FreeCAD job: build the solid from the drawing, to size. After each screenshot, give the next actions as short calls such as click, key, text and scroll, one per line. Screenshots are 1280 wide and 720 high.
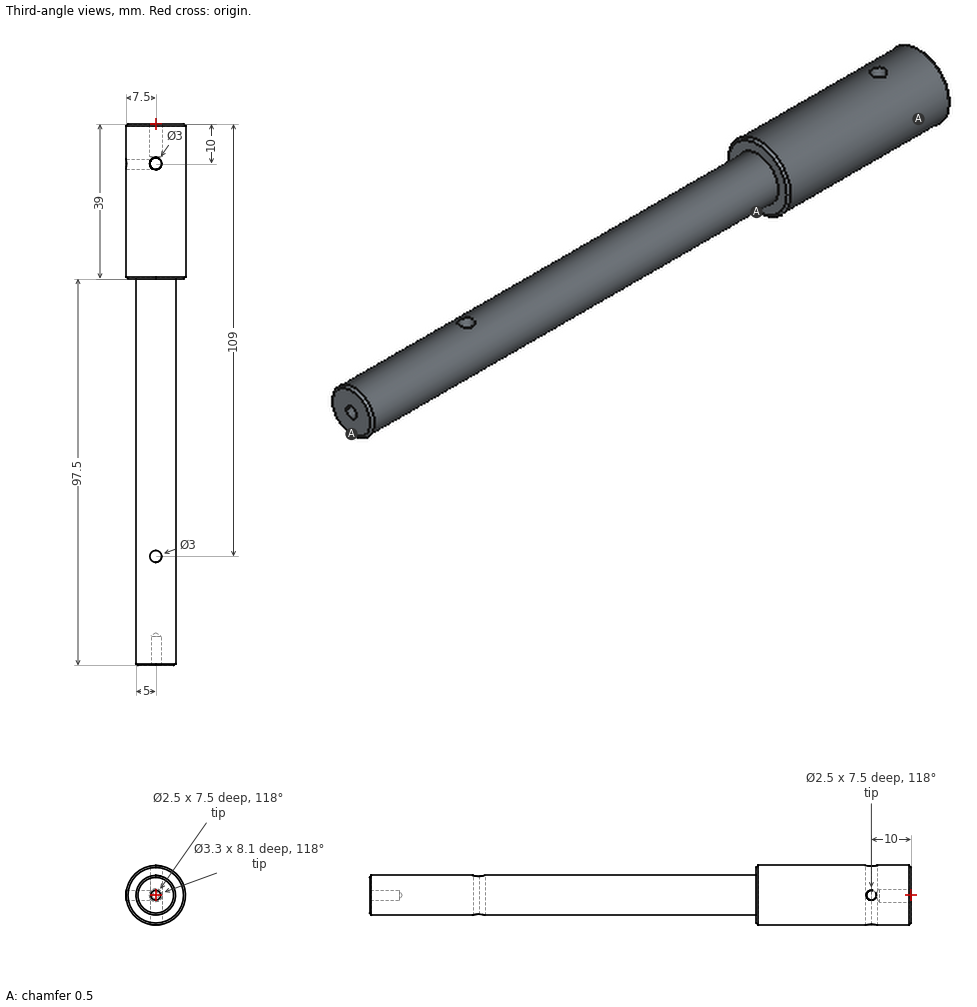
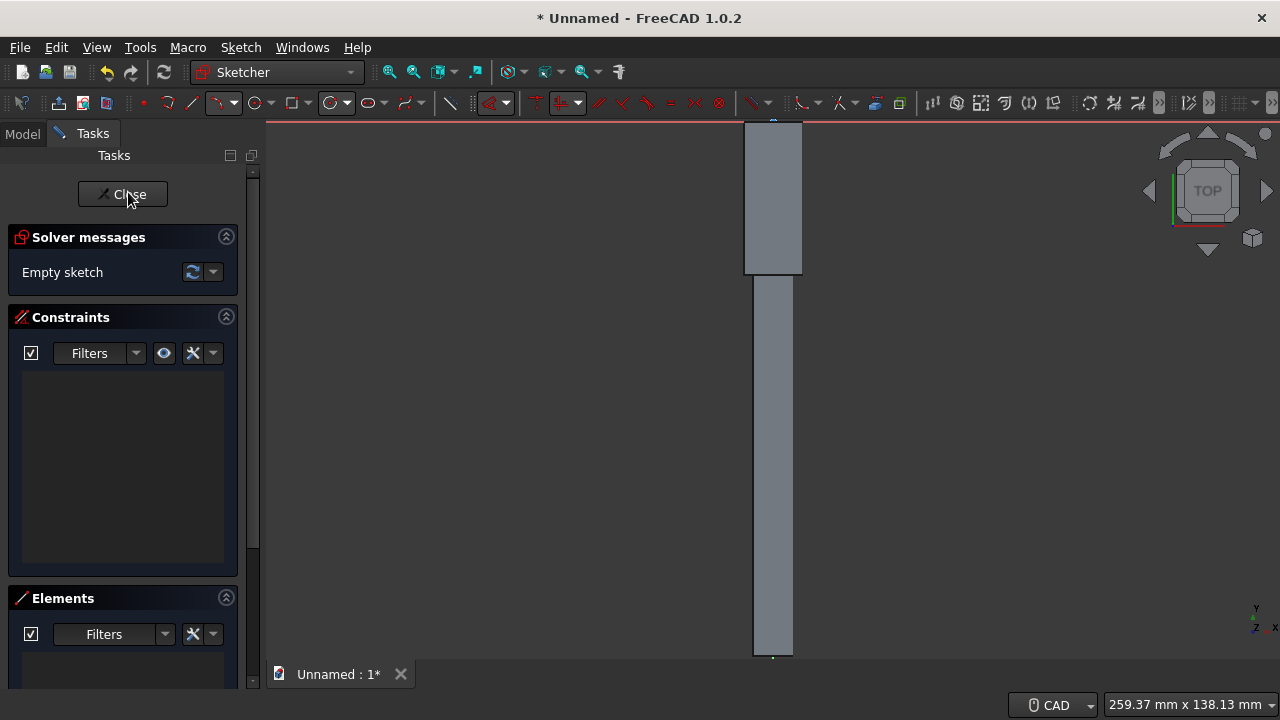
click(108, 104)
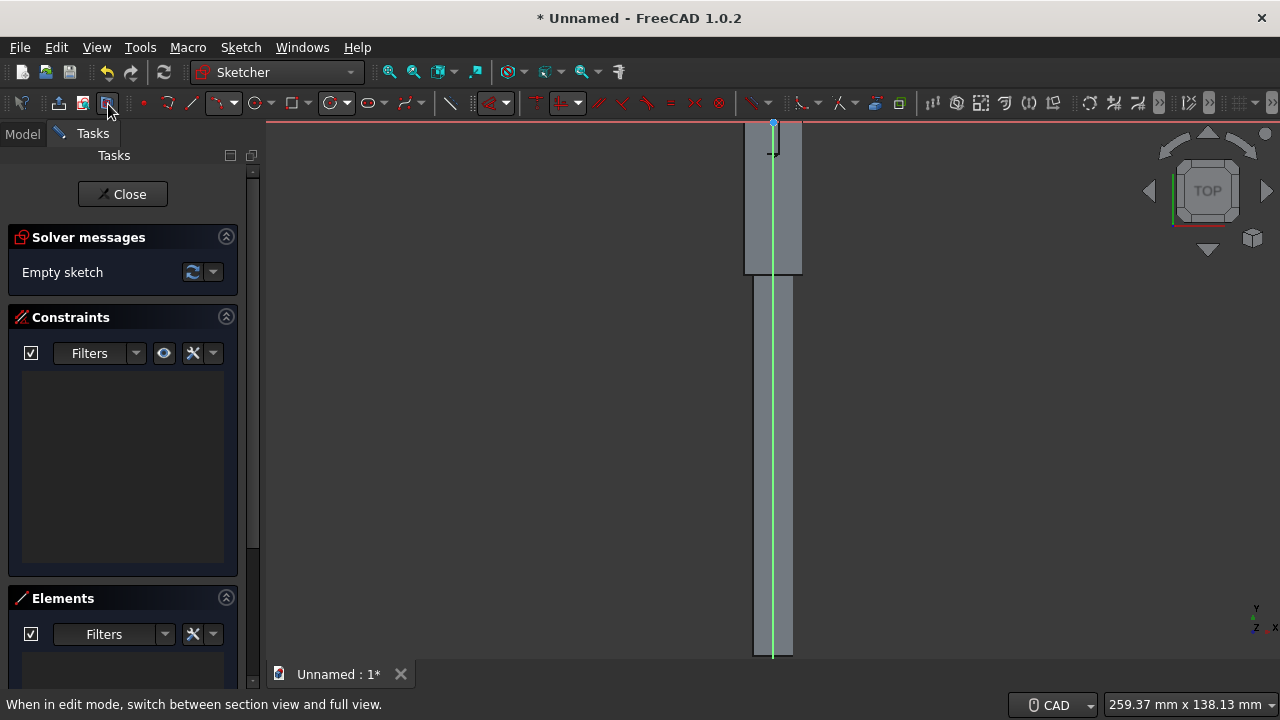
scroll(777, 149, up, 15)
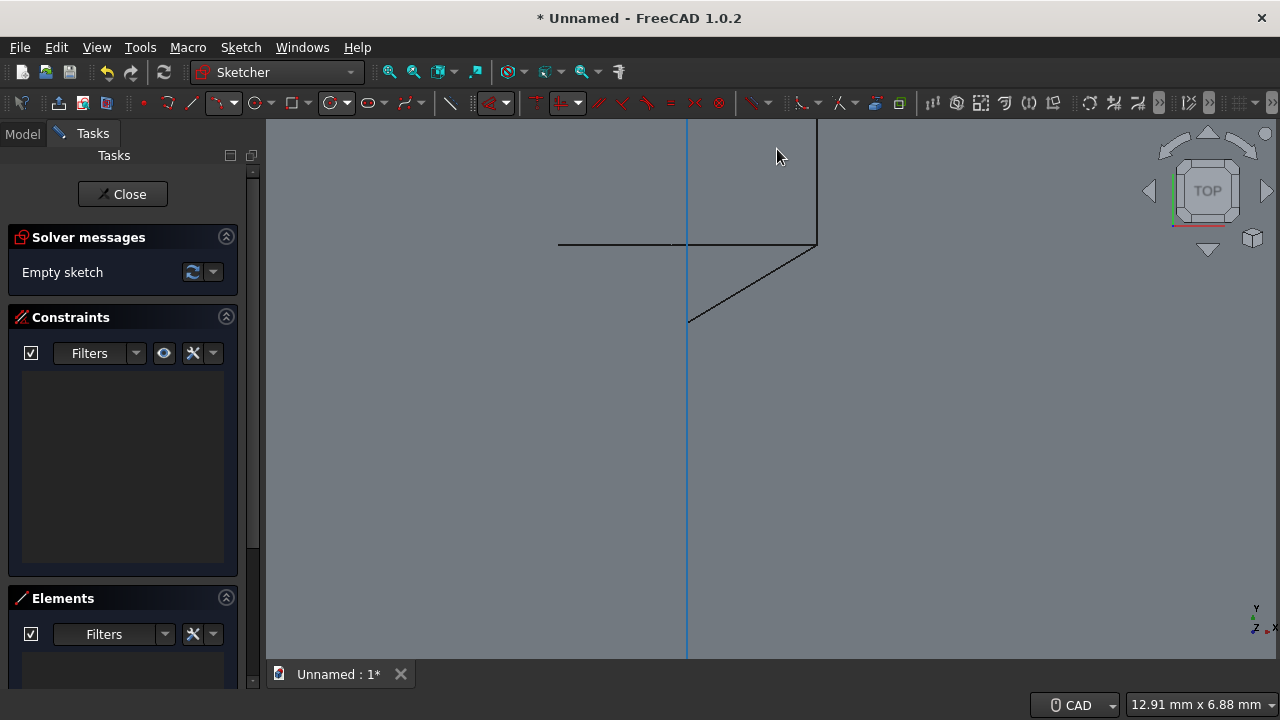
scroll(652, 406, up, 2)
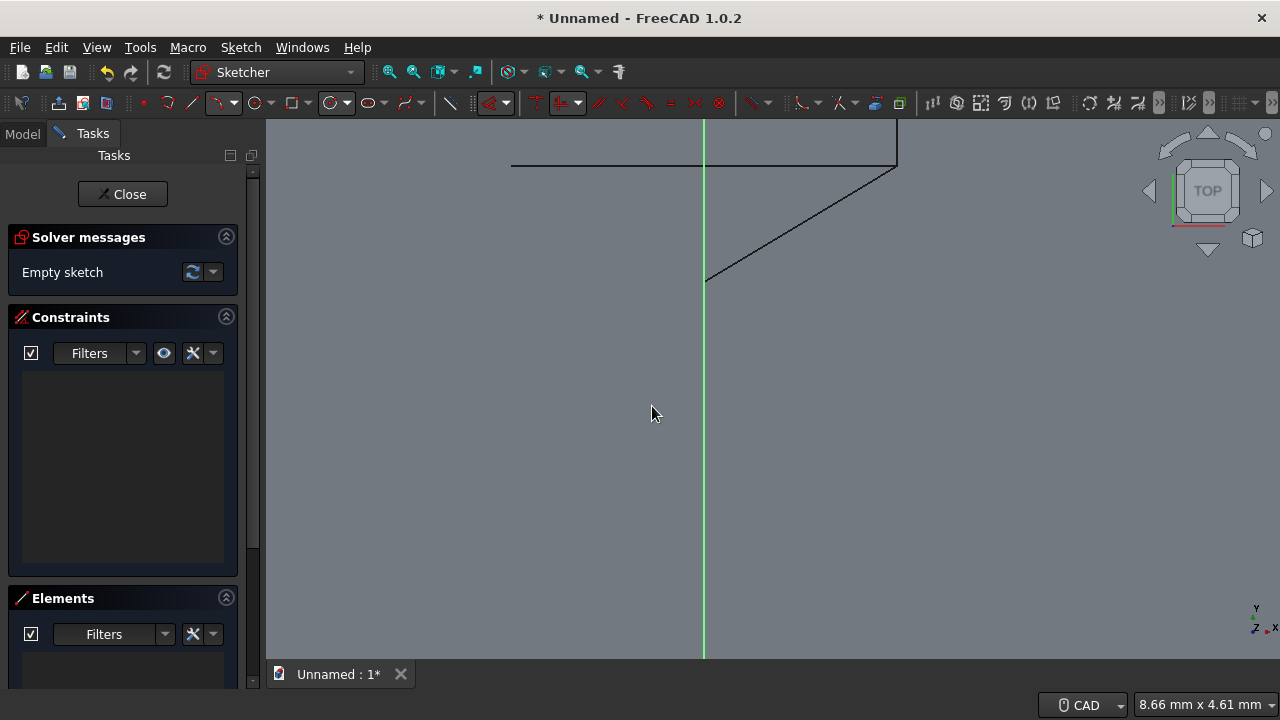
click(256, 104)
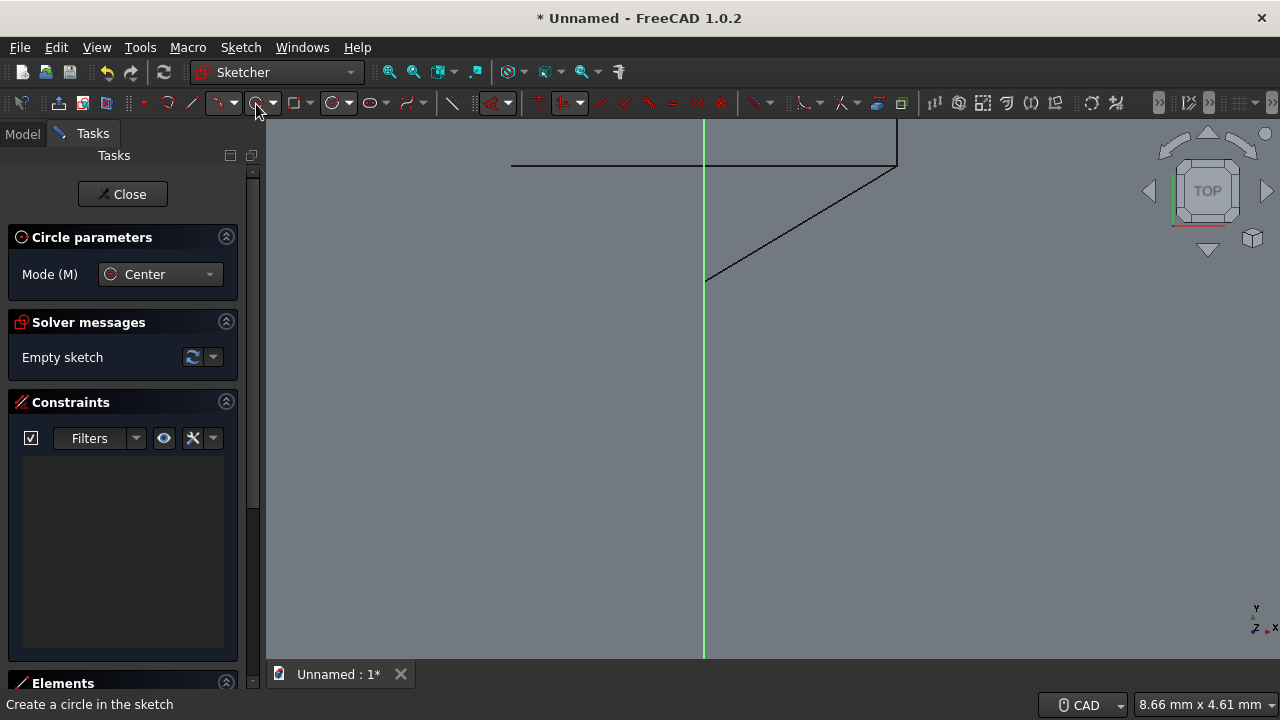
click(704, 389)
click(828, 264)
key(Escape)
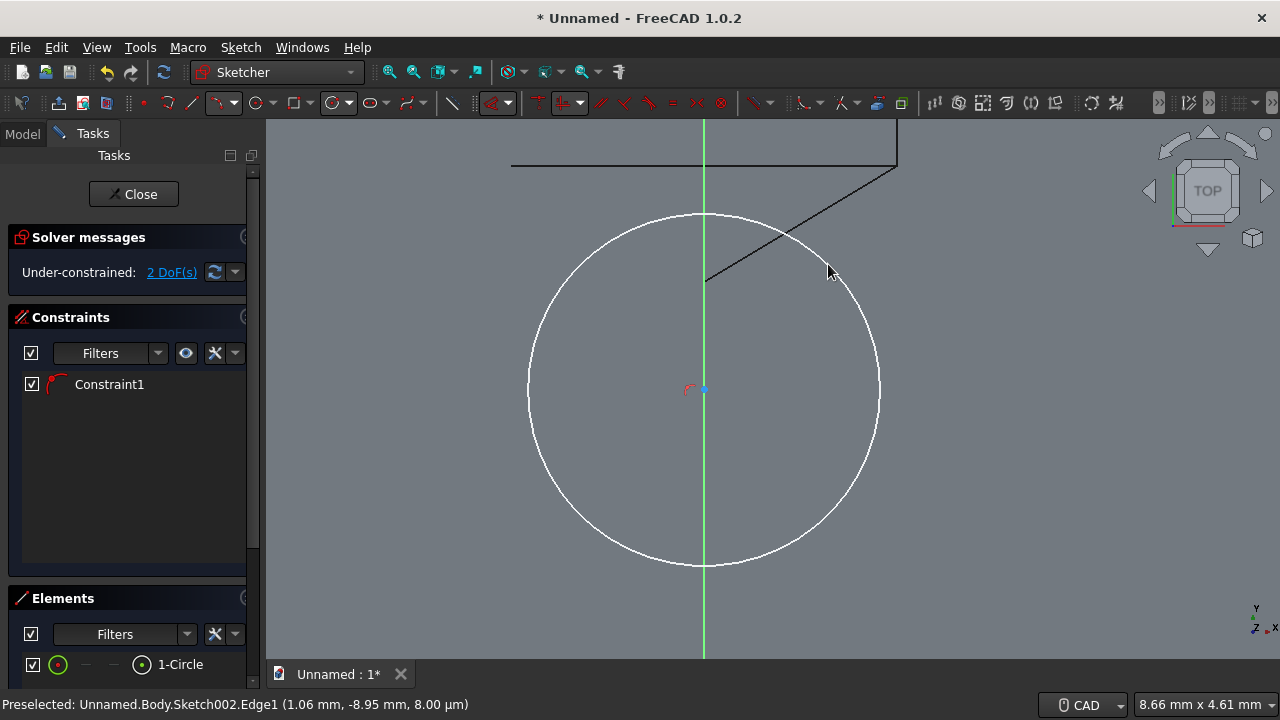
click(828, 265)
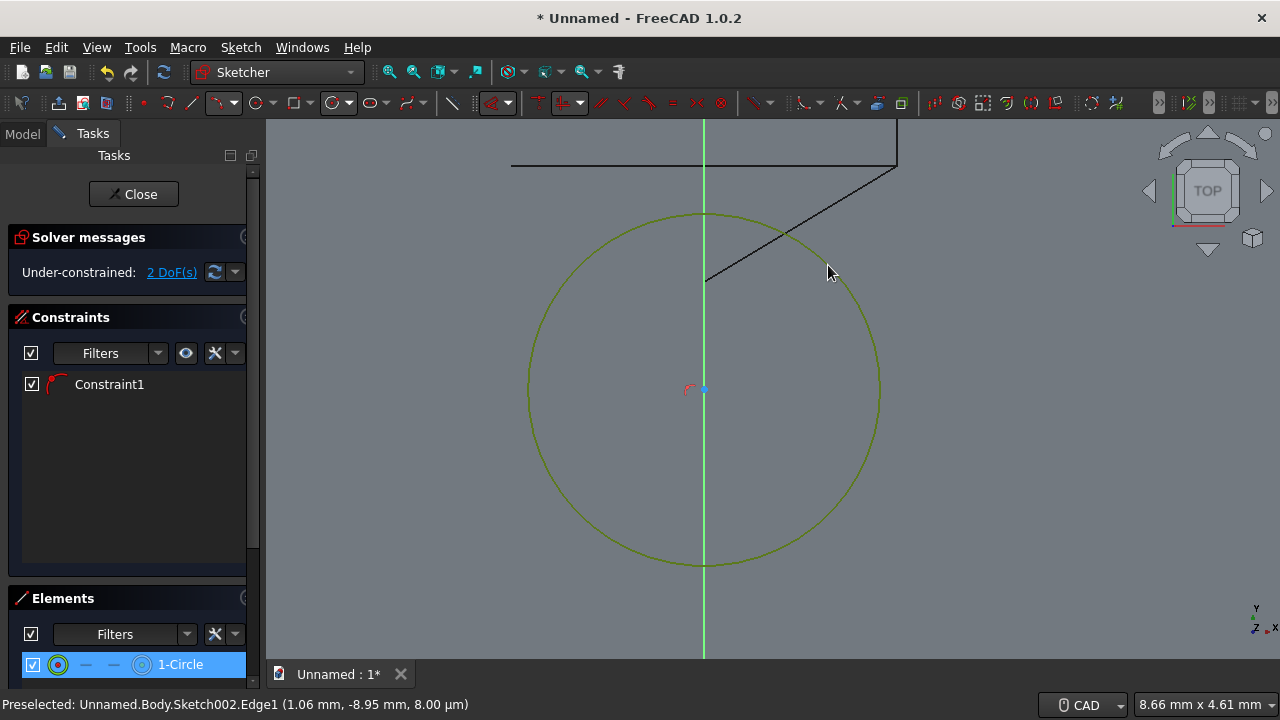
key(k)
key(o)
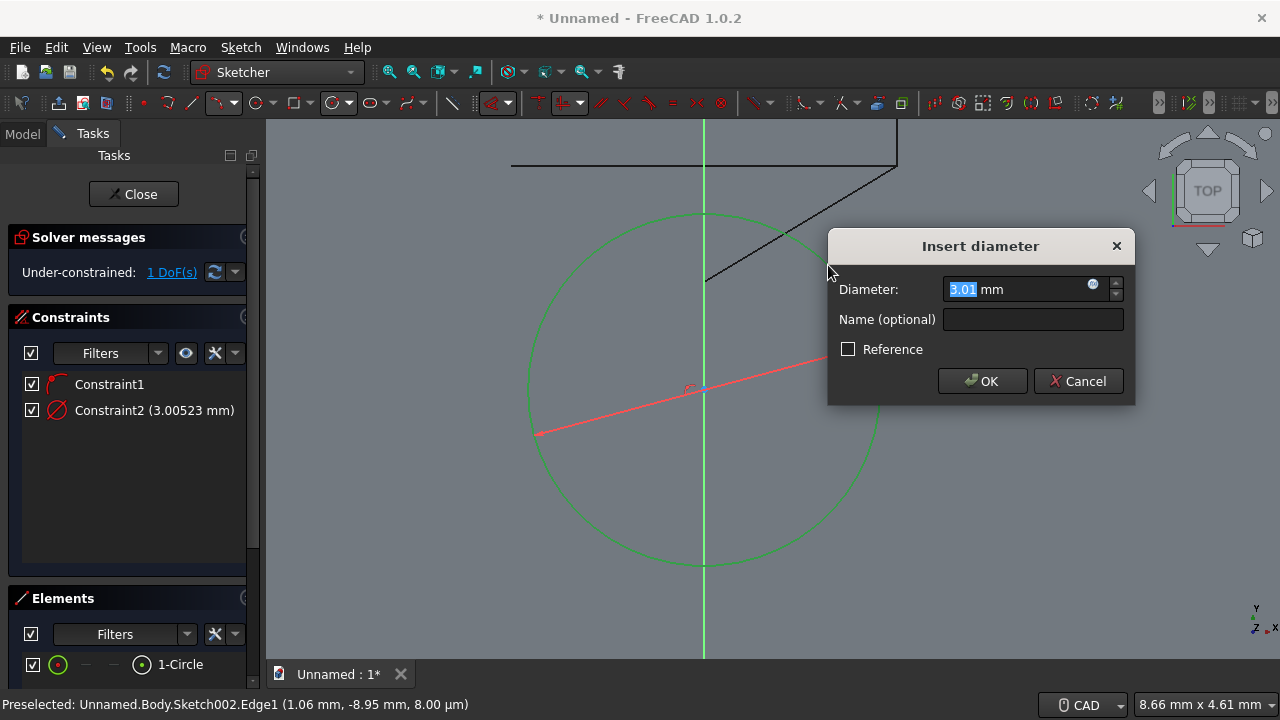
text(3)
key(Return)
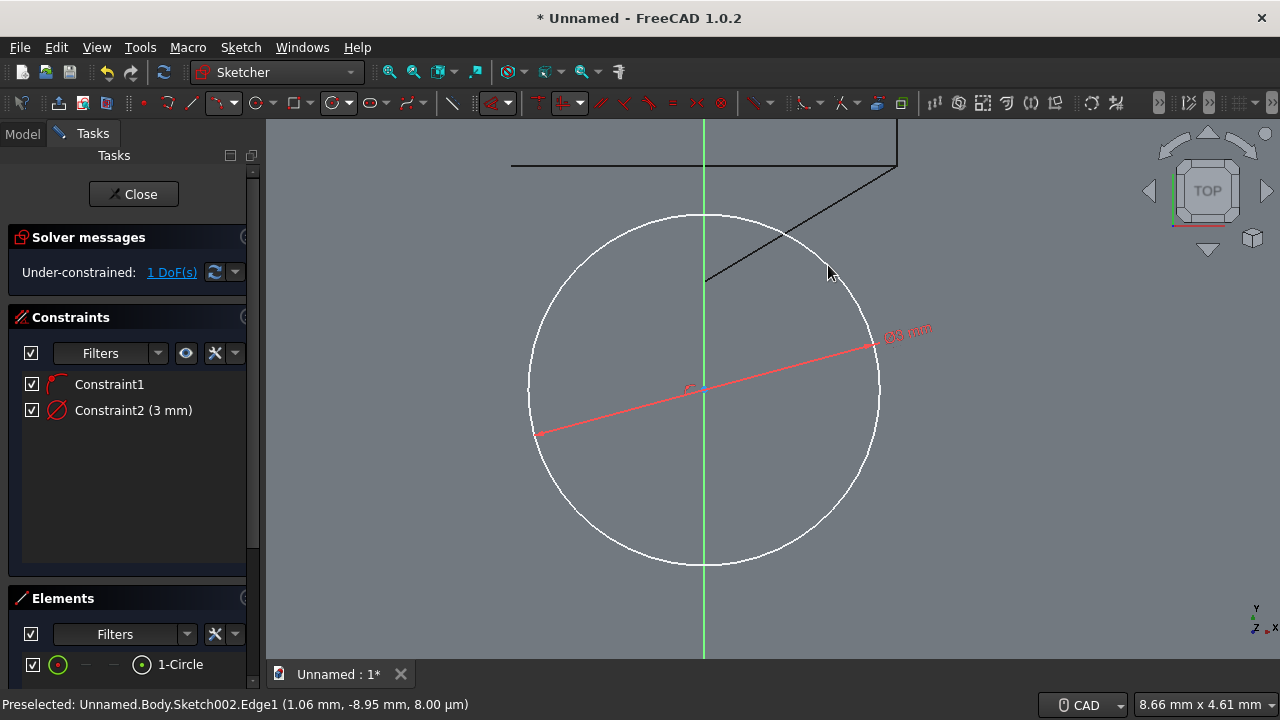
click(704, 390)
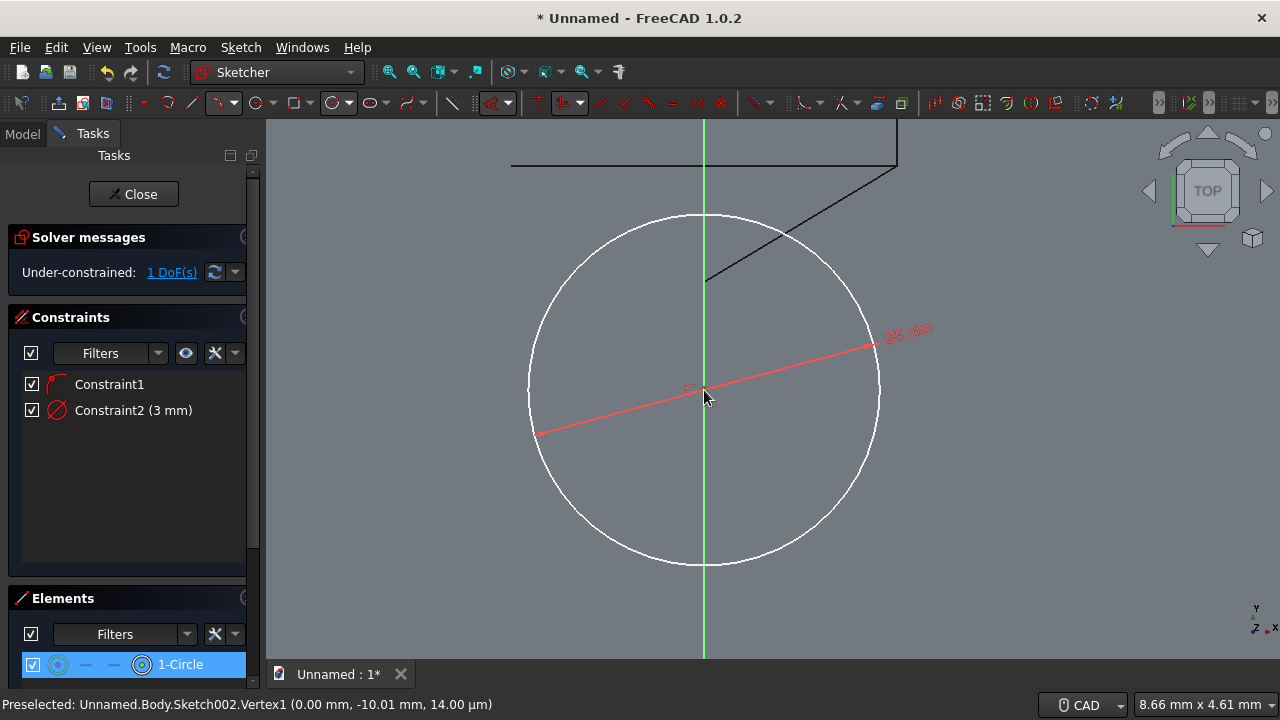
key(i)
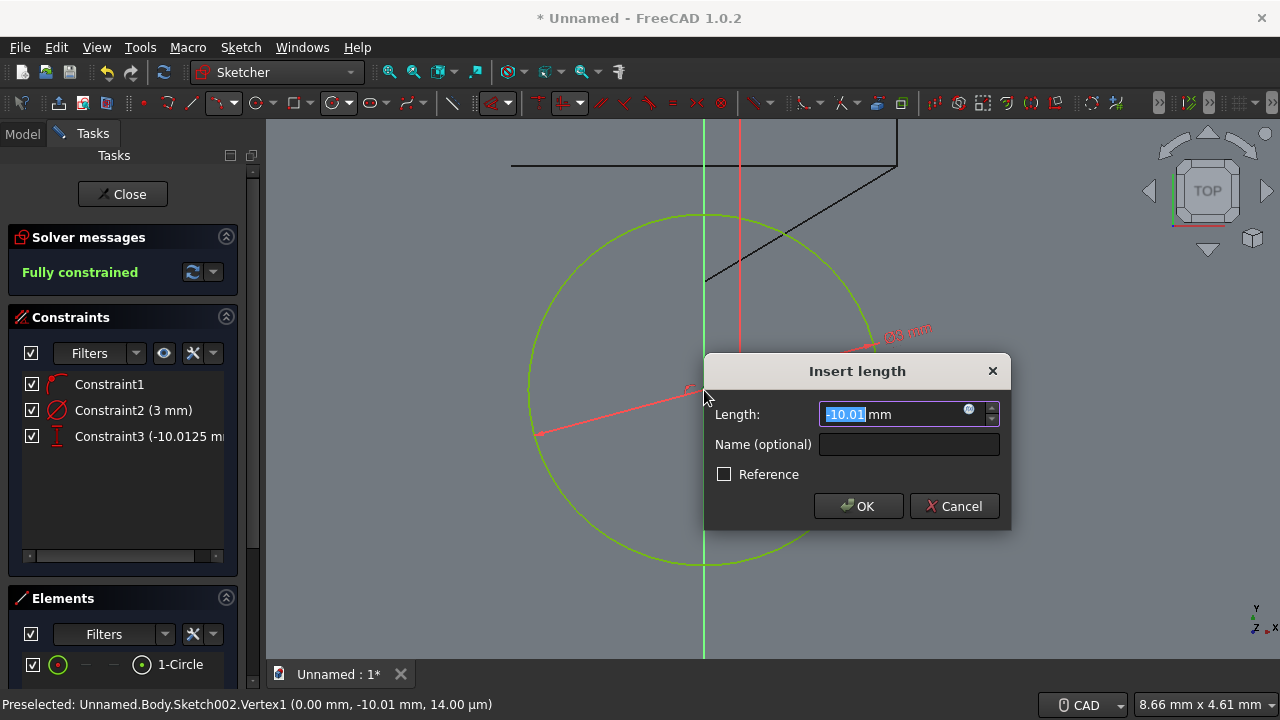
text(-10)
key(Return)